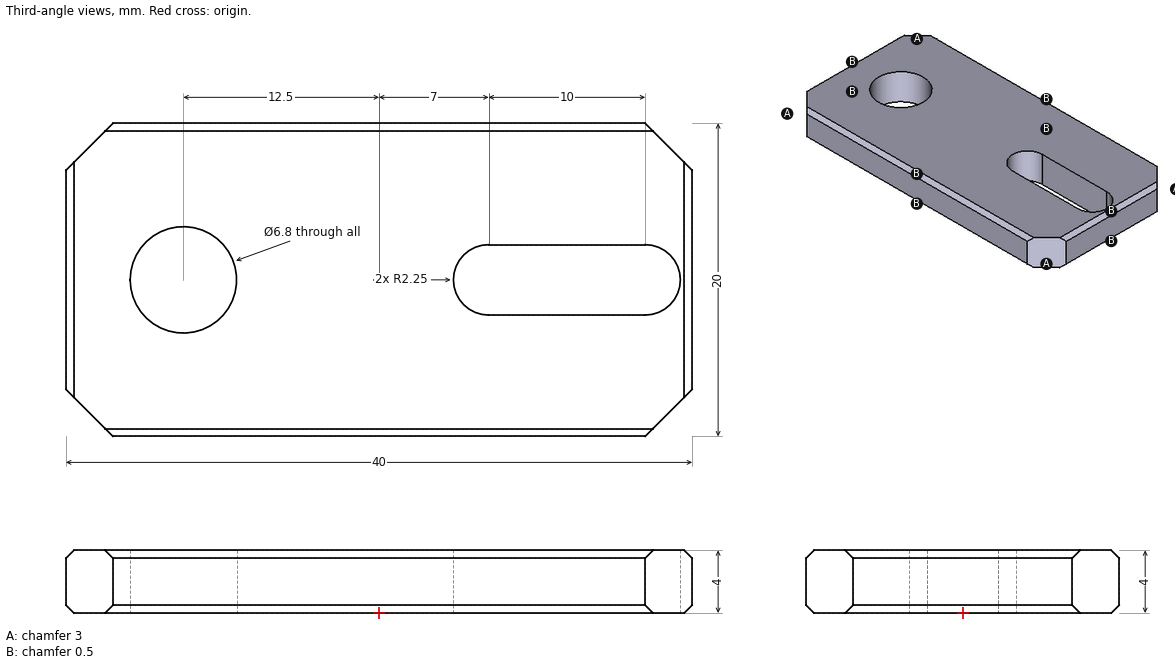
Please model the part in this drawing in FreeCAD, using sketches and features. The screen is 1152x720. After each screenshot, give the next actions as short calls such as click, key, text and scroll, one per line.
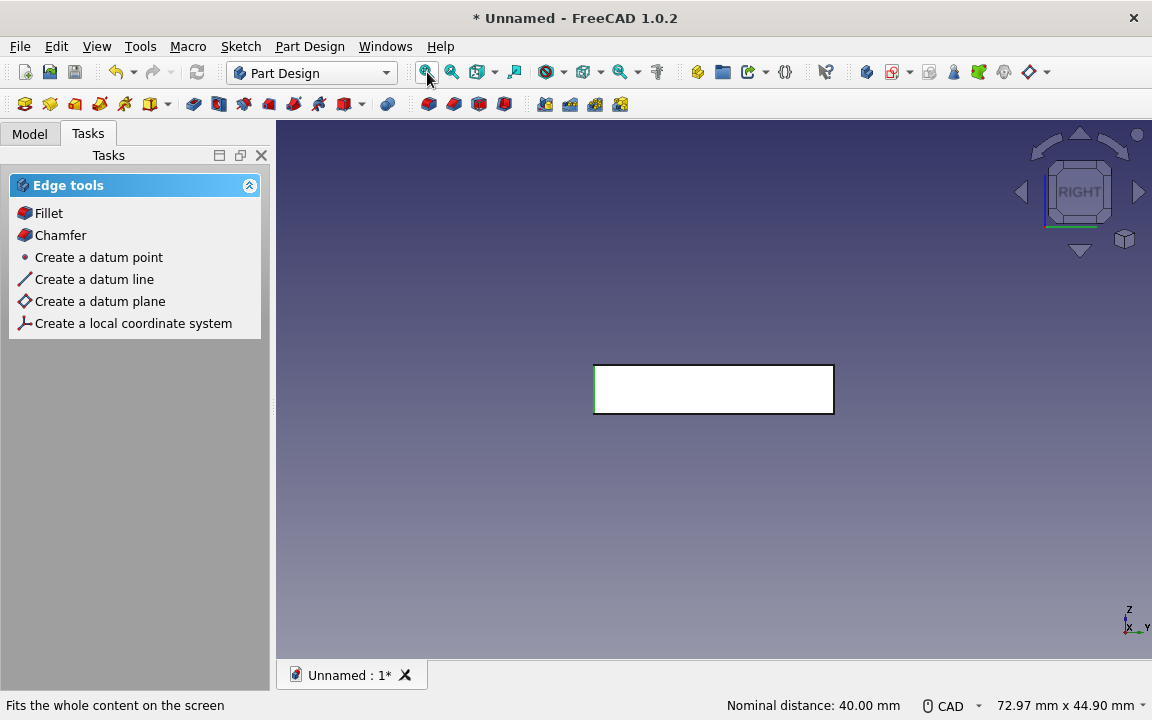
click(834, 388, ctrl)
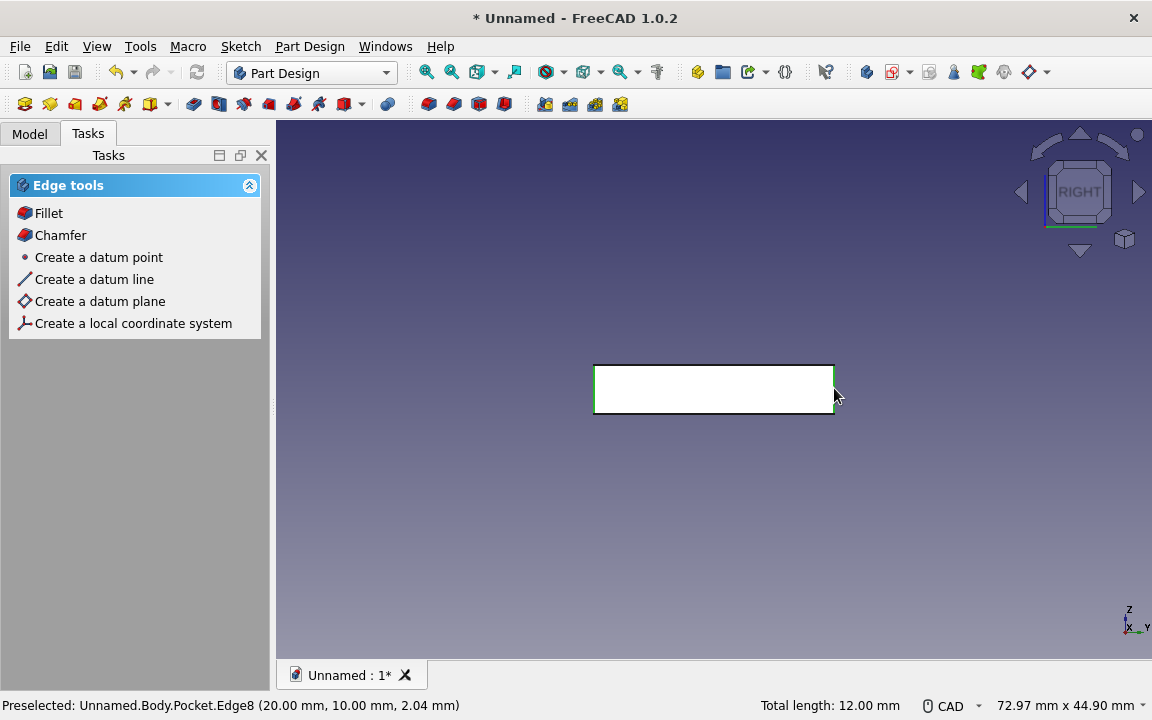
key(5)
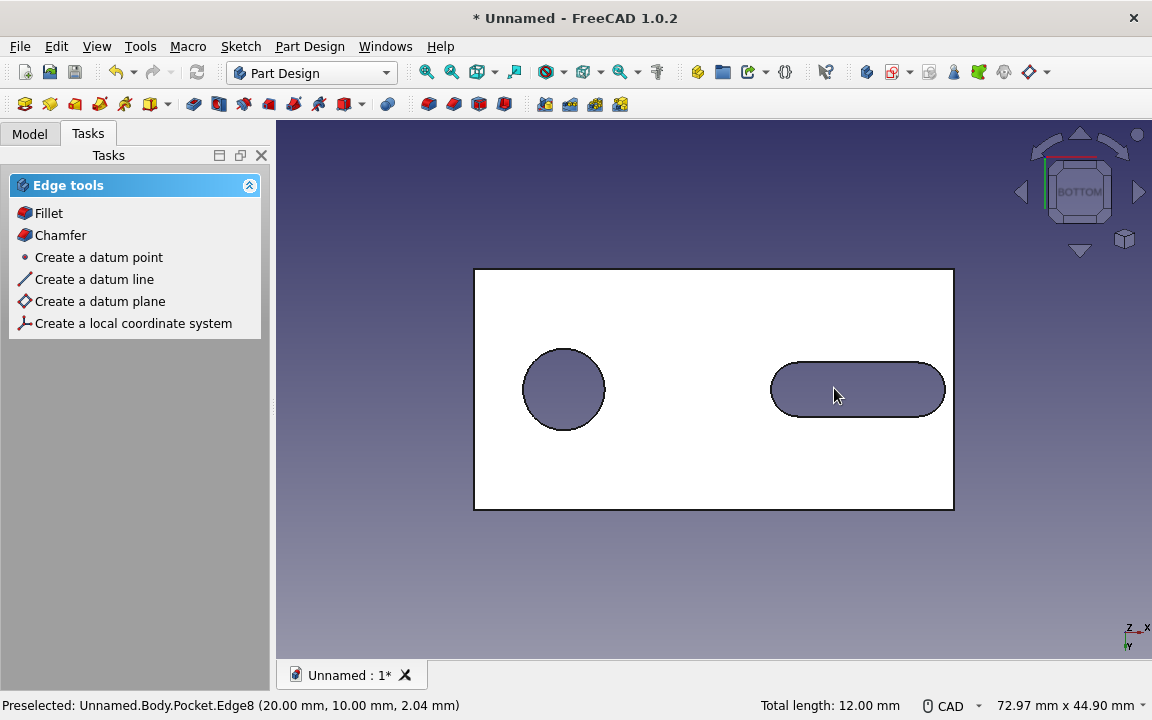
key(4)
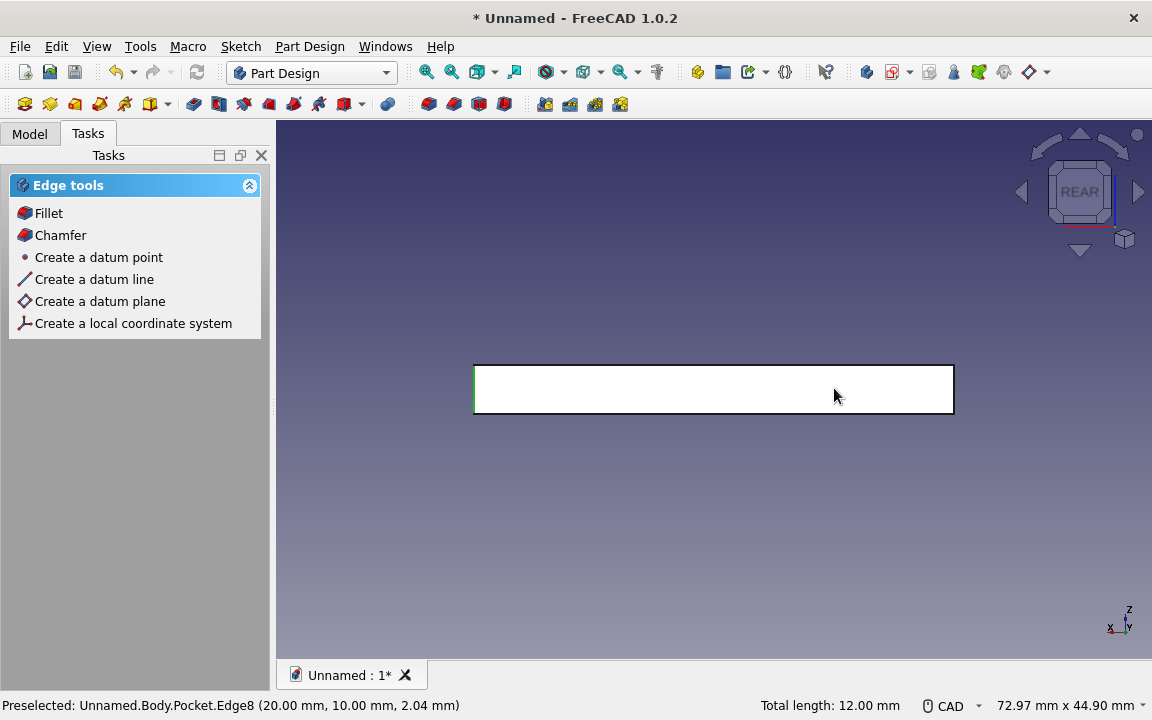
click(954, 388, ctrl)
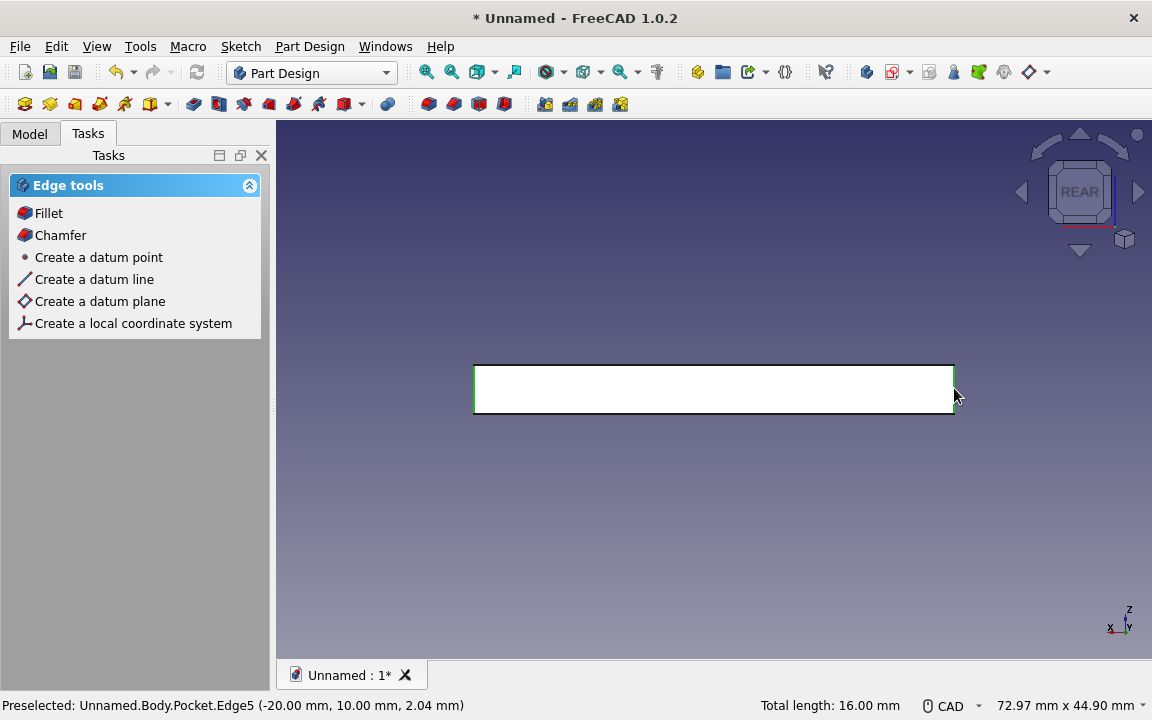
click(454, 104)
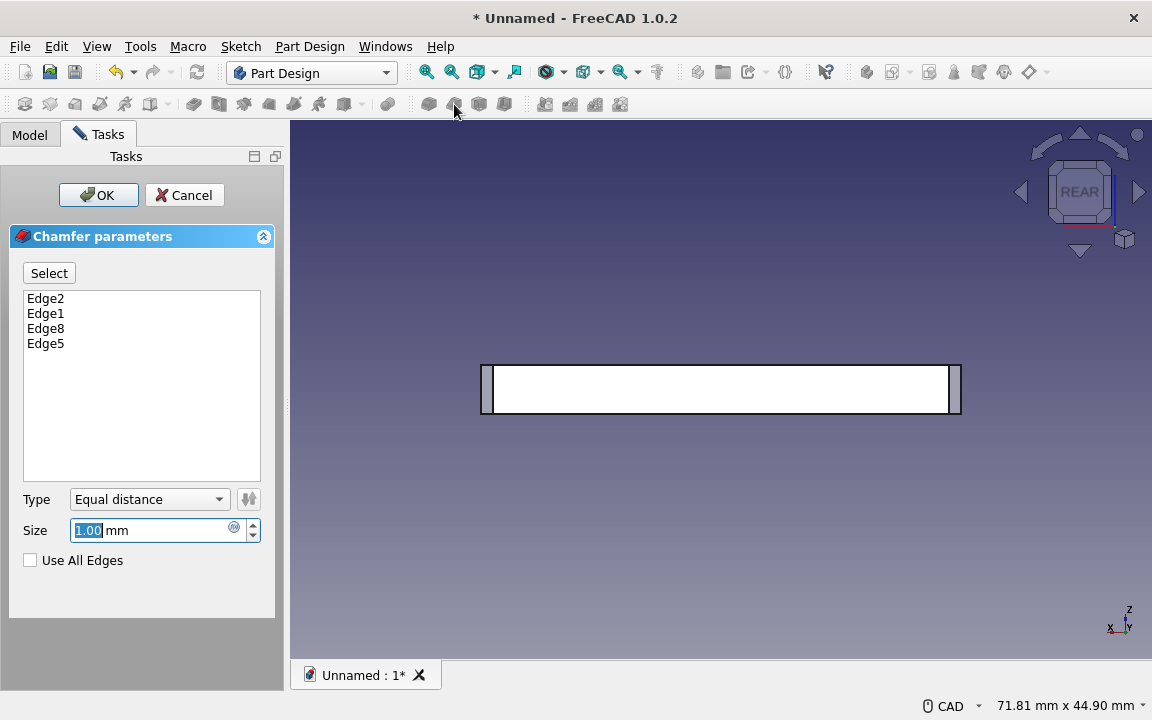
text(3)
key(Tab)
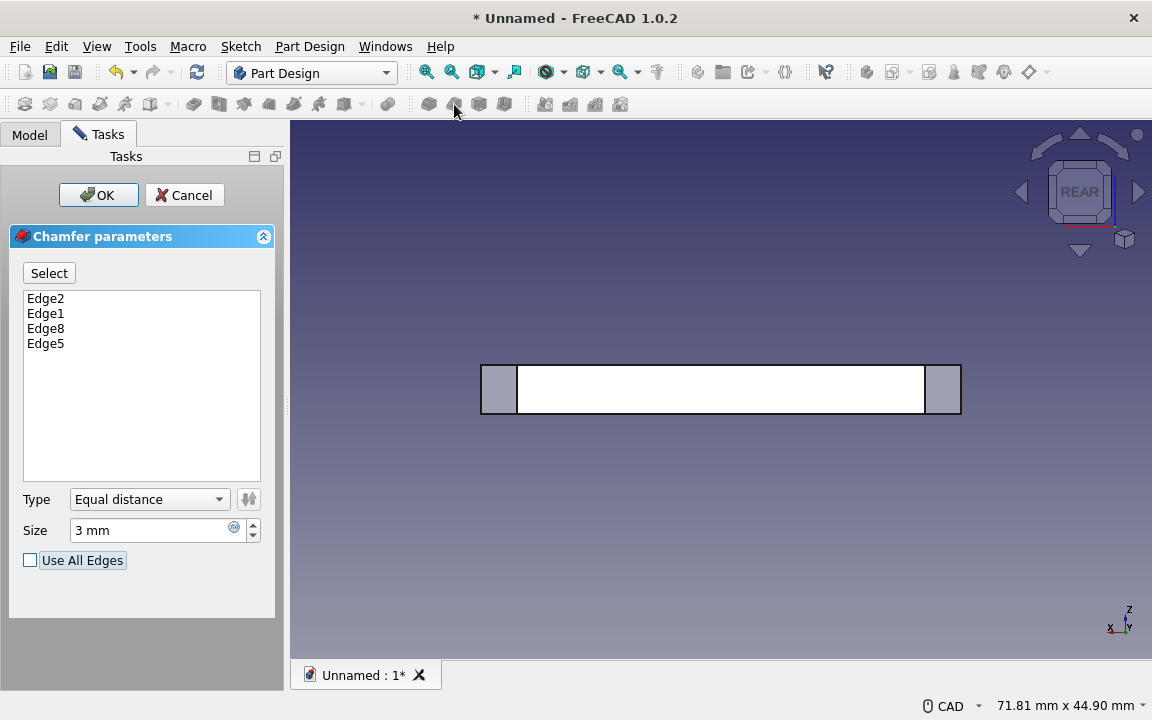
click(99, 195)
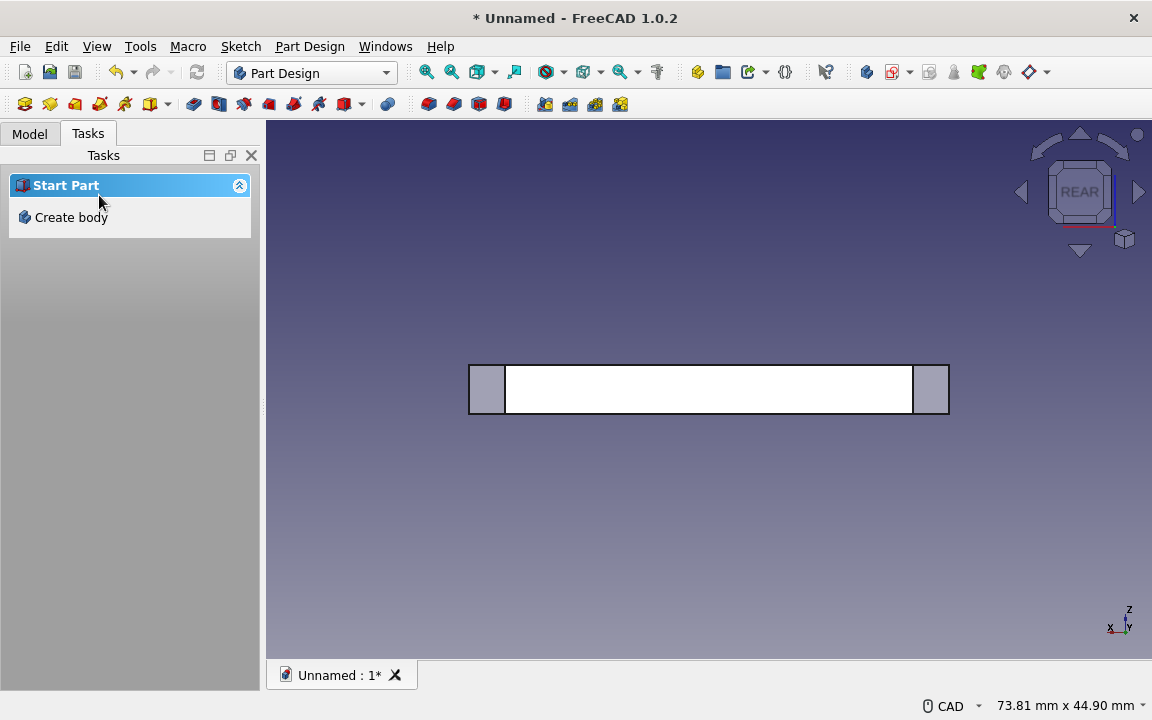
click(709, 413)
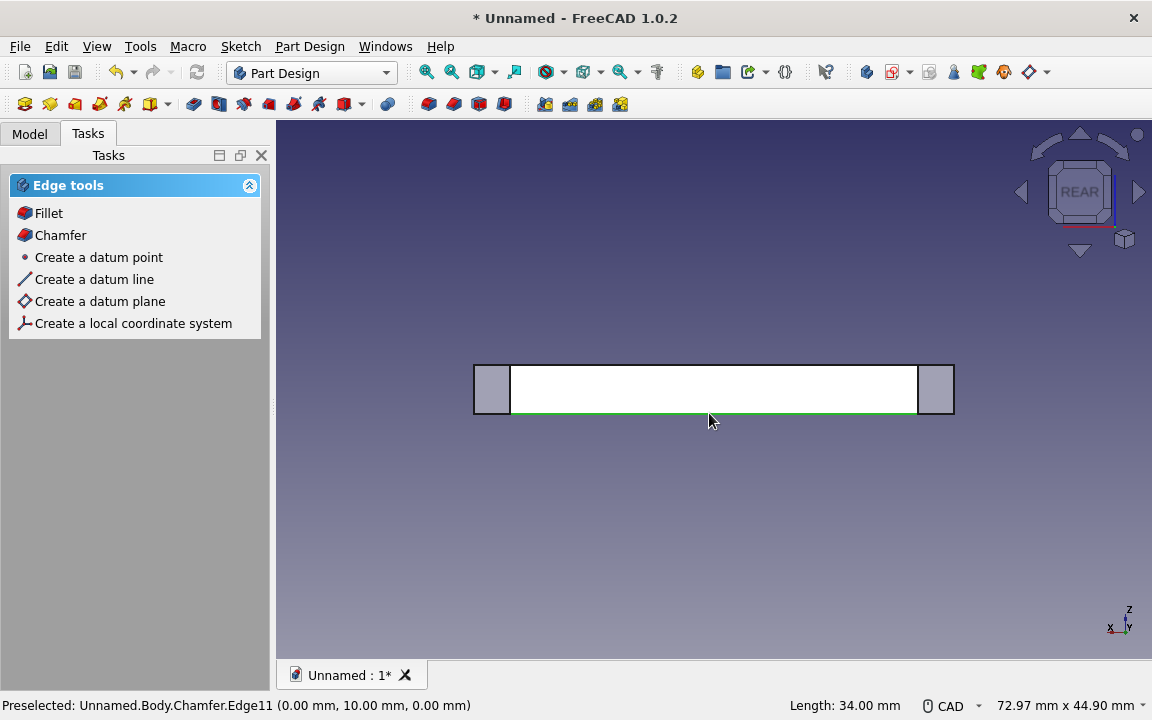
click(714, 364, ctrl)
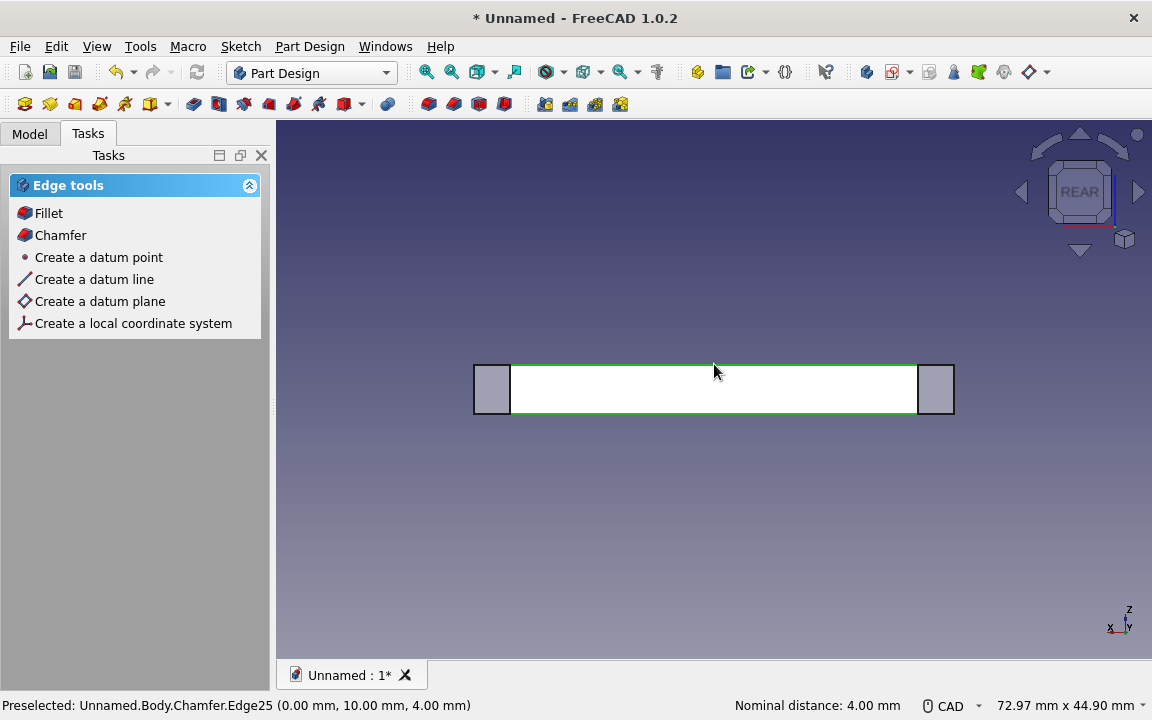
key(0)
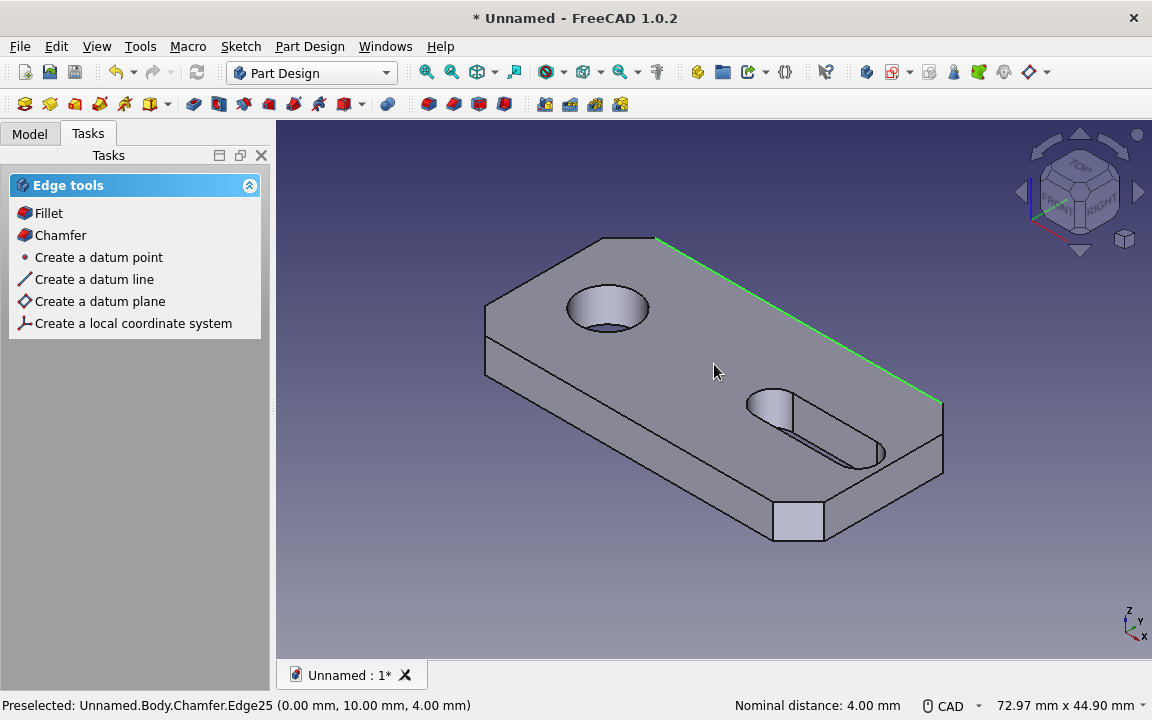
click(884, 467, ctrl)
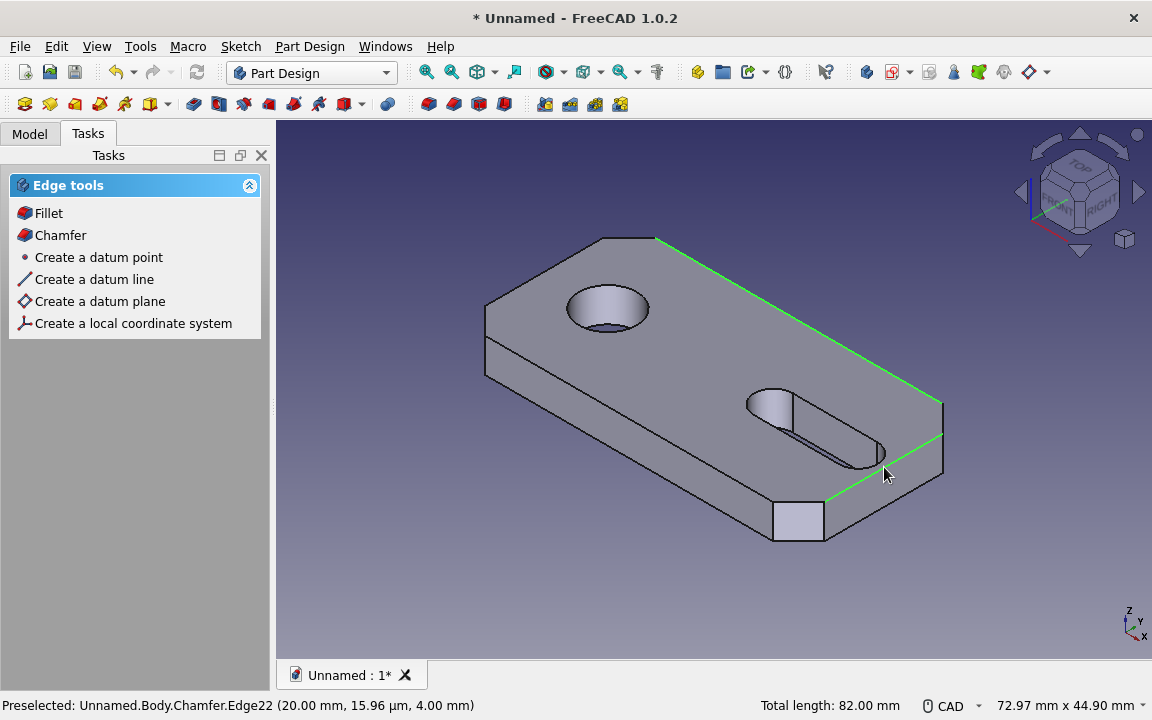
click(629, 418, ctrl)